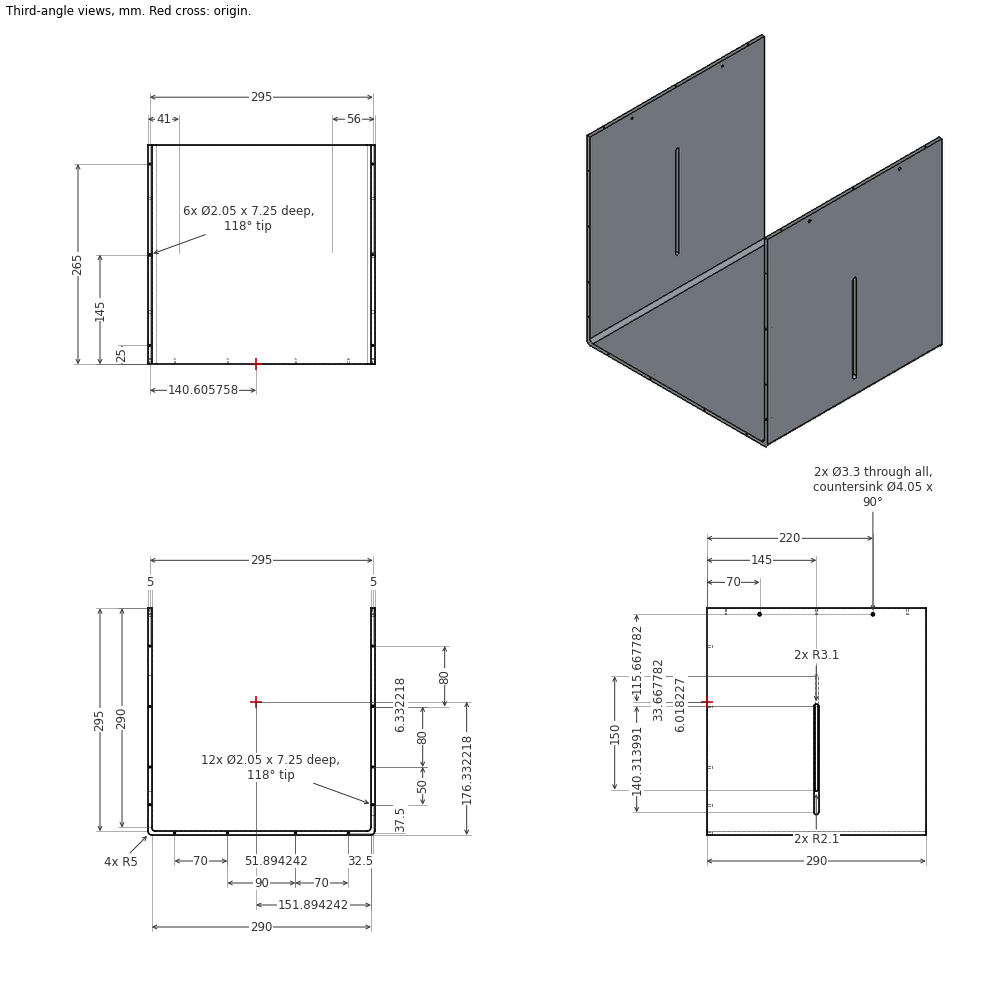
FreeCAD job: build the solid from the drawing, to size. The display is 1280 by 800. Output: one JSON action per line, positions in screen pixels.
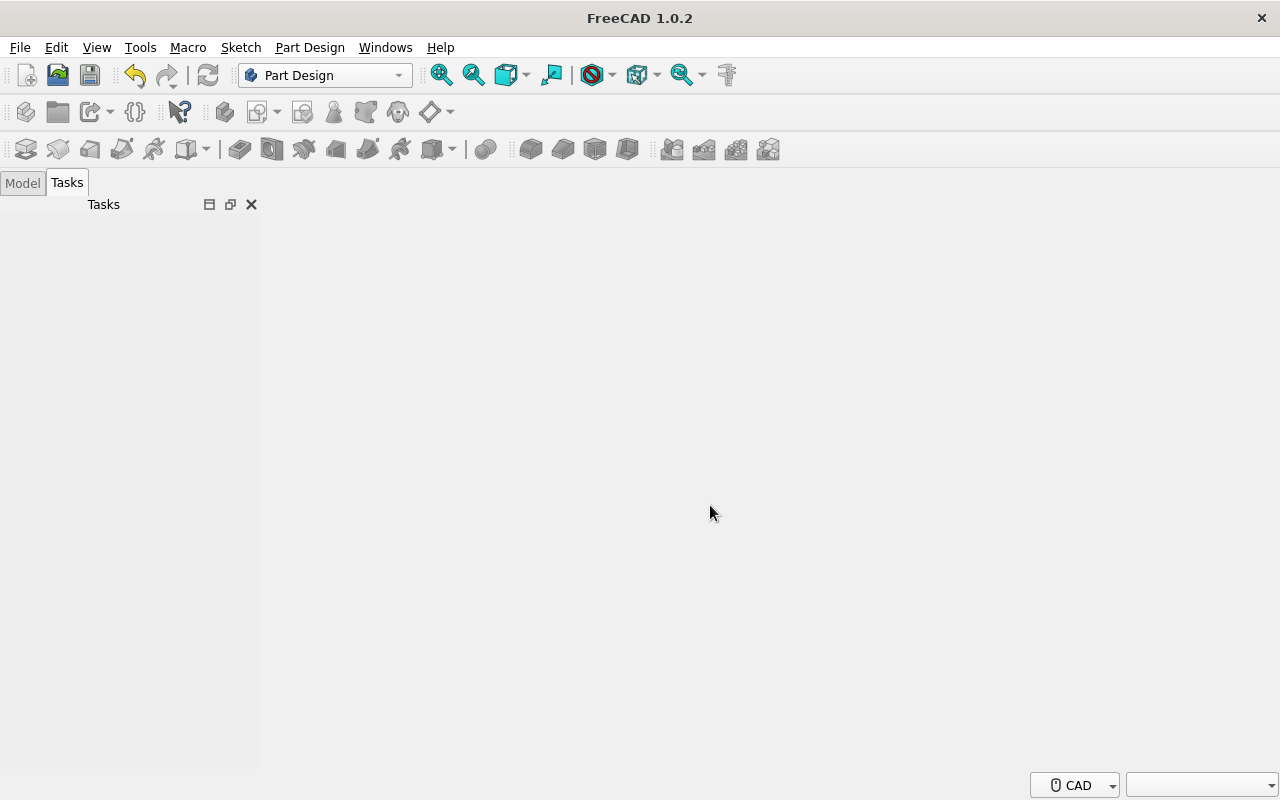
{"action": "left_click", "coordinate": [26, 76]}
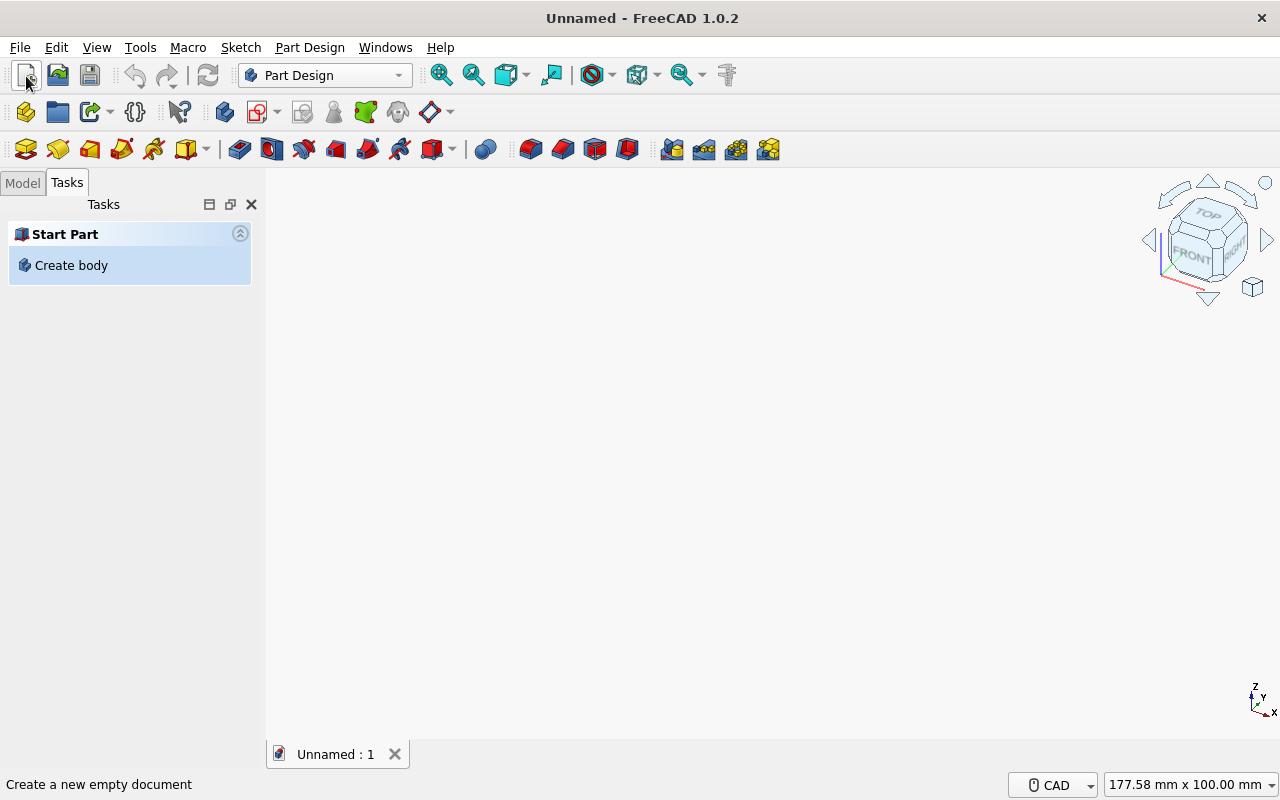
{"action": "left_click", "coordinate": [258, 112]}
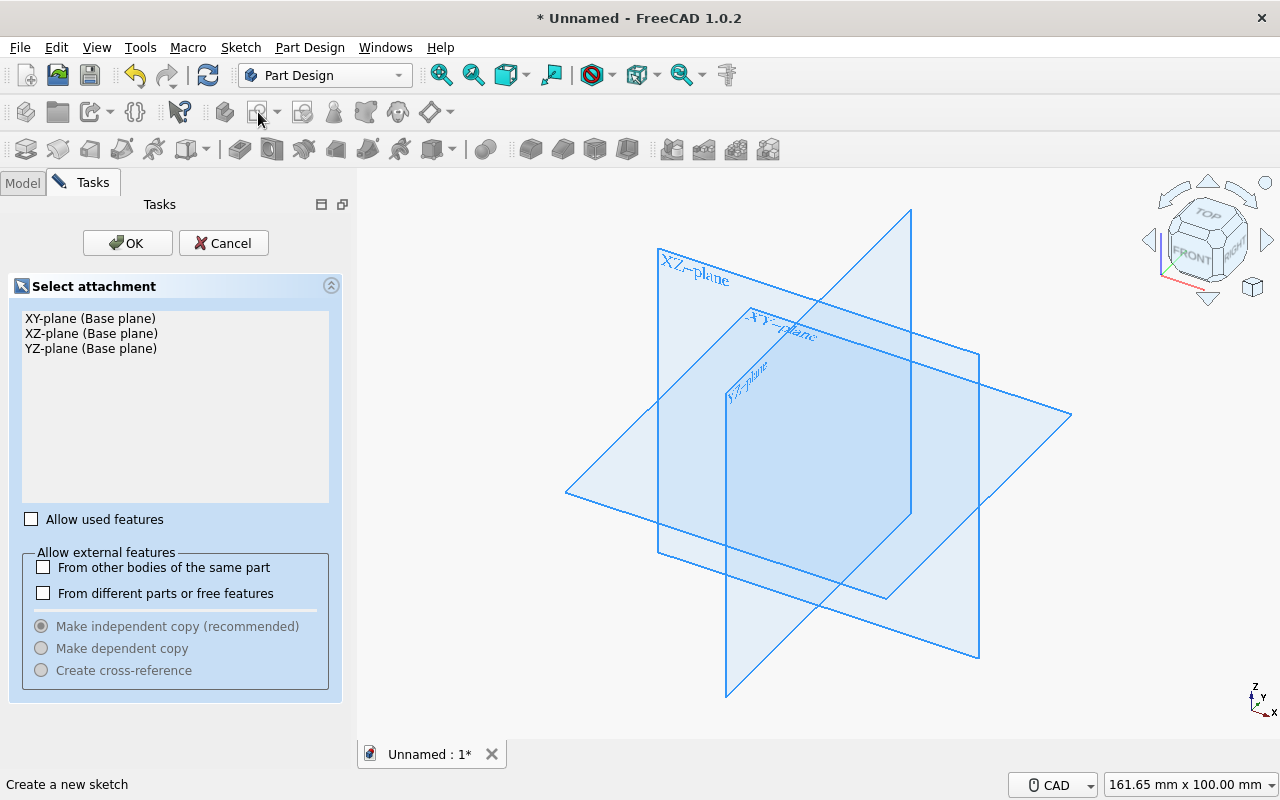
{"action": "left_click", "coordinate": [82, 334]}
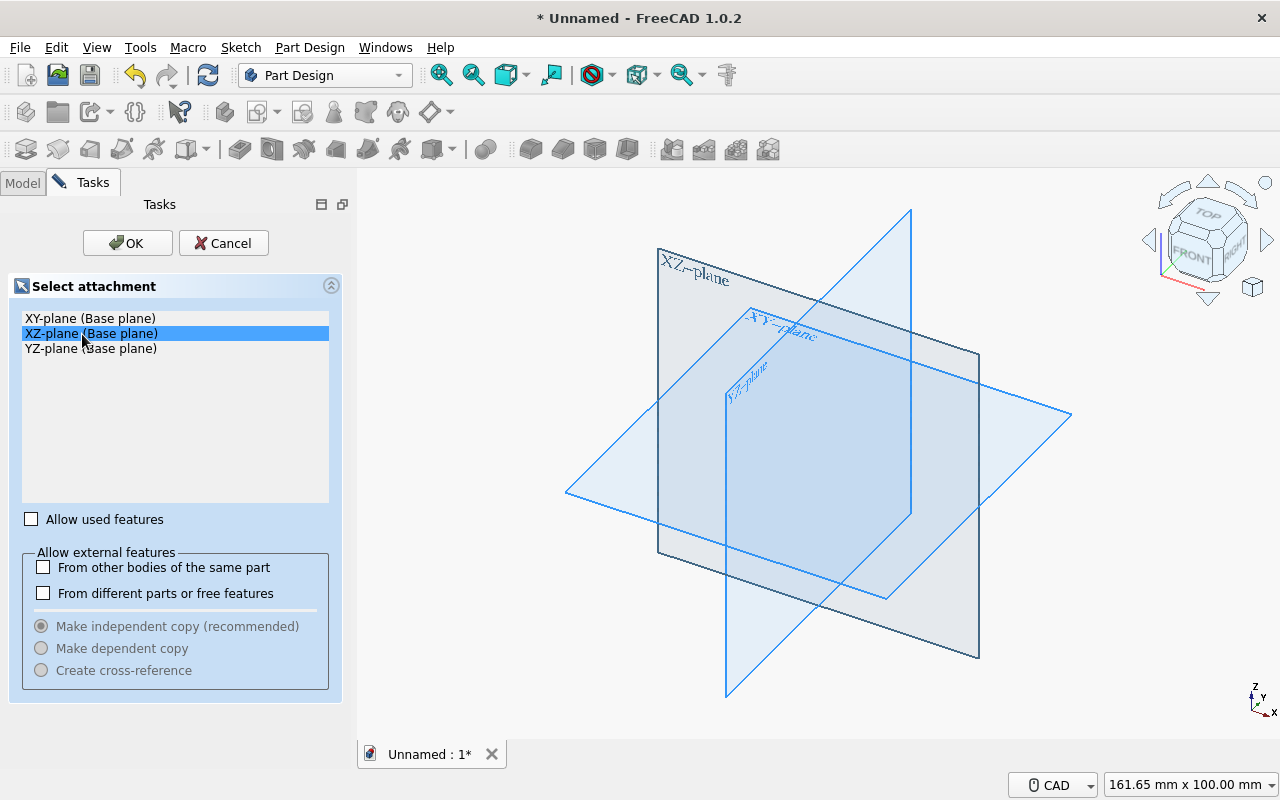
{"action": "left_click", "coordinate": [128, 243]}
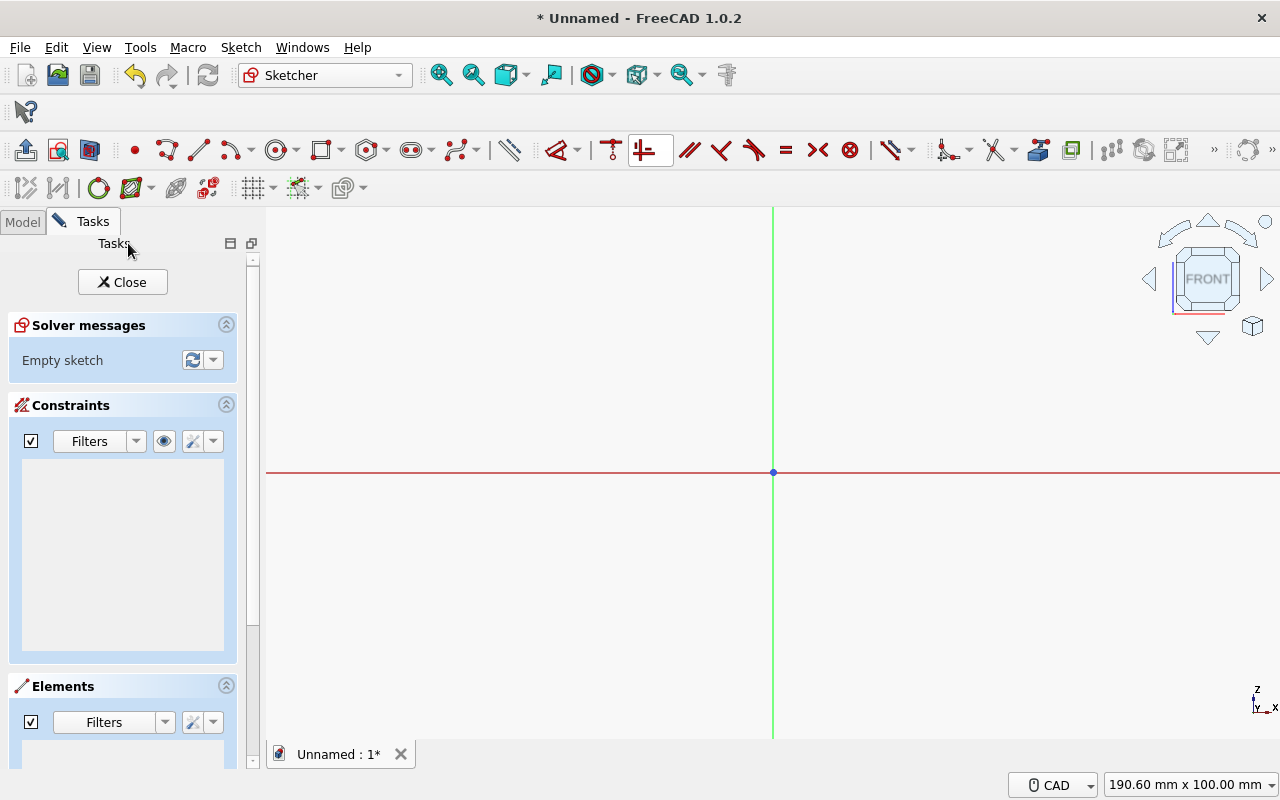
{"action": "scroll", "coordinate": [678, 438], "scroll_direction": "down", "scroll_amount": 8}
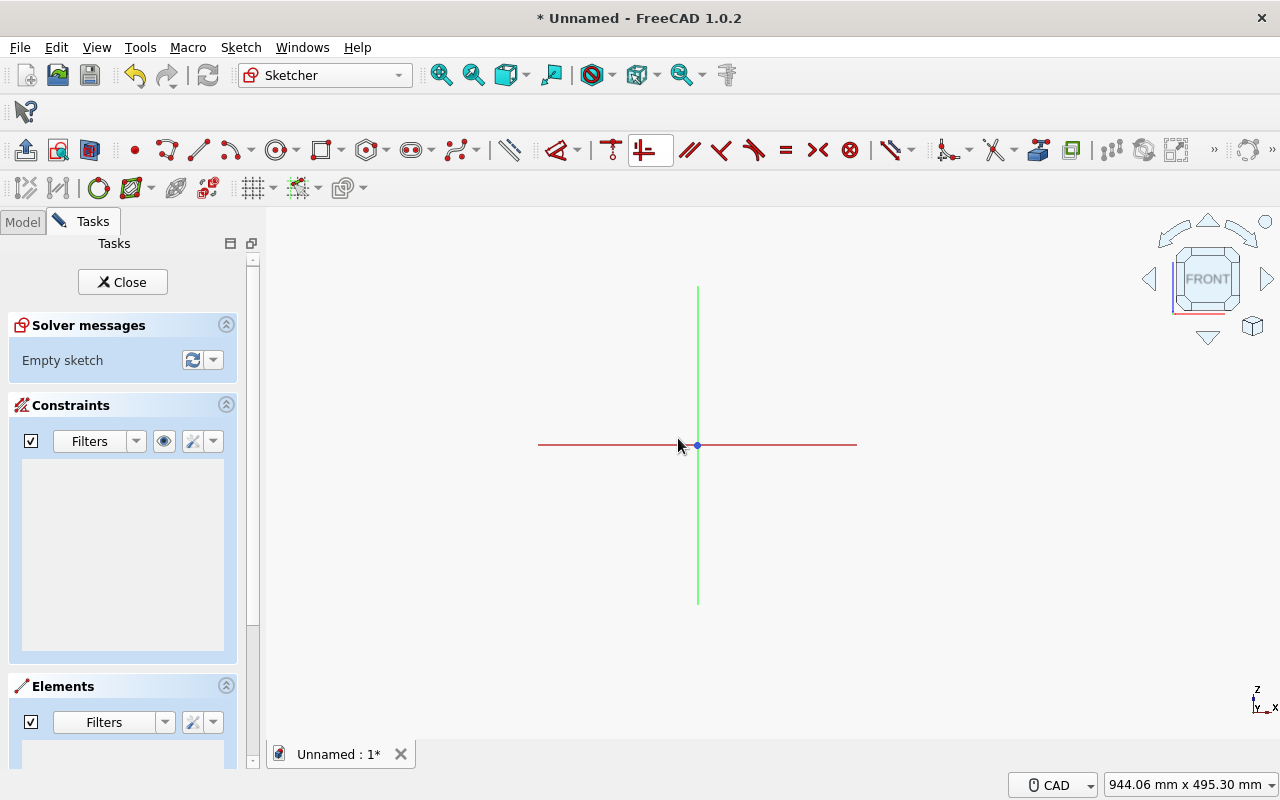
{"action": "left_click", "coordinate": [200, 150]}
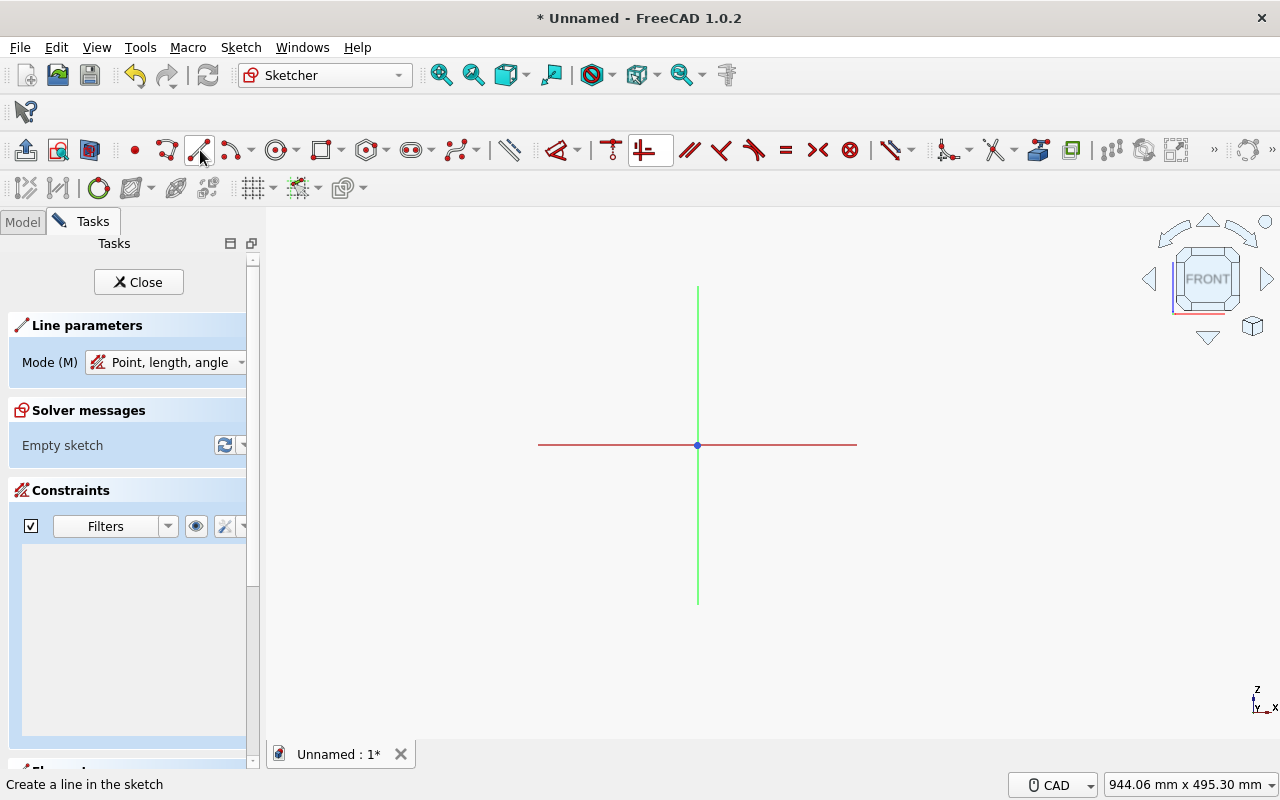
{"action": "left_click", "coordinate": [861, 635]}
{"action": "left_click", "coordinate": [549, 635]}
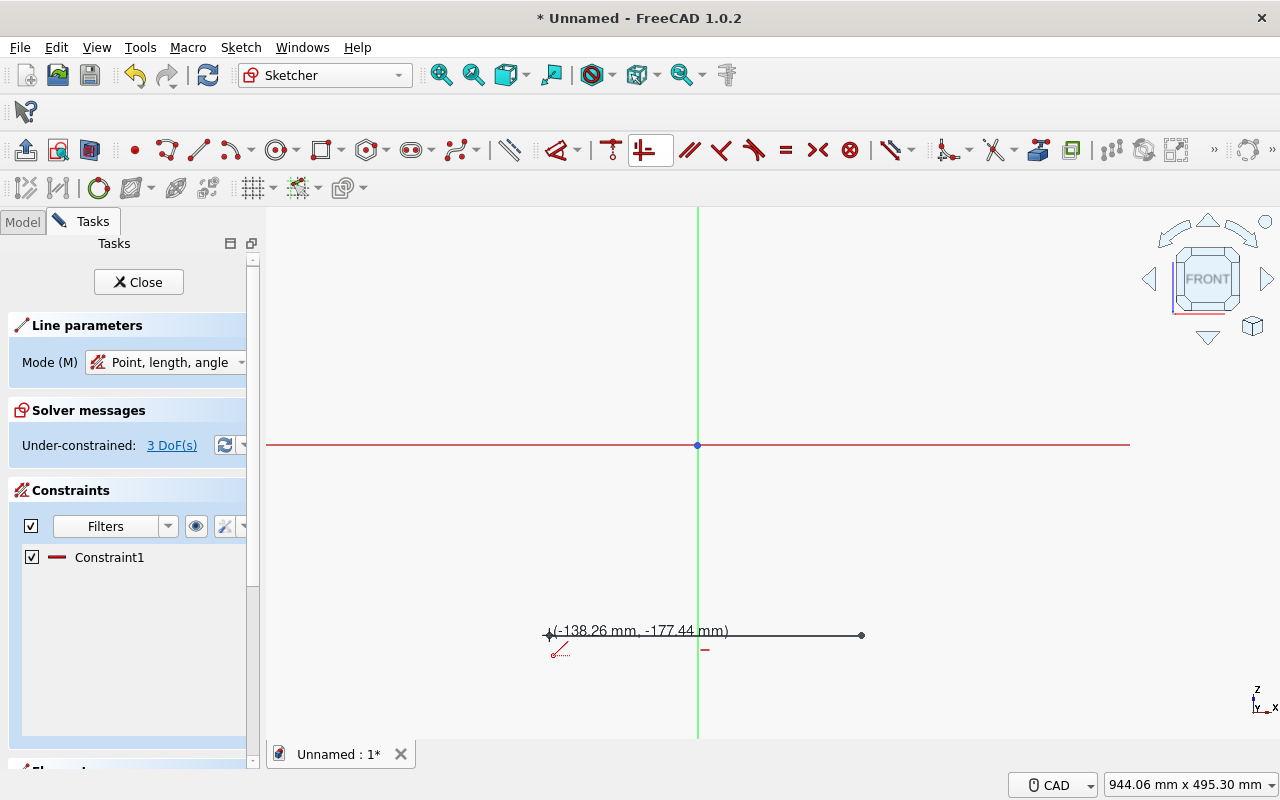
{"action": "left_click", "coordinate": [168, 150]}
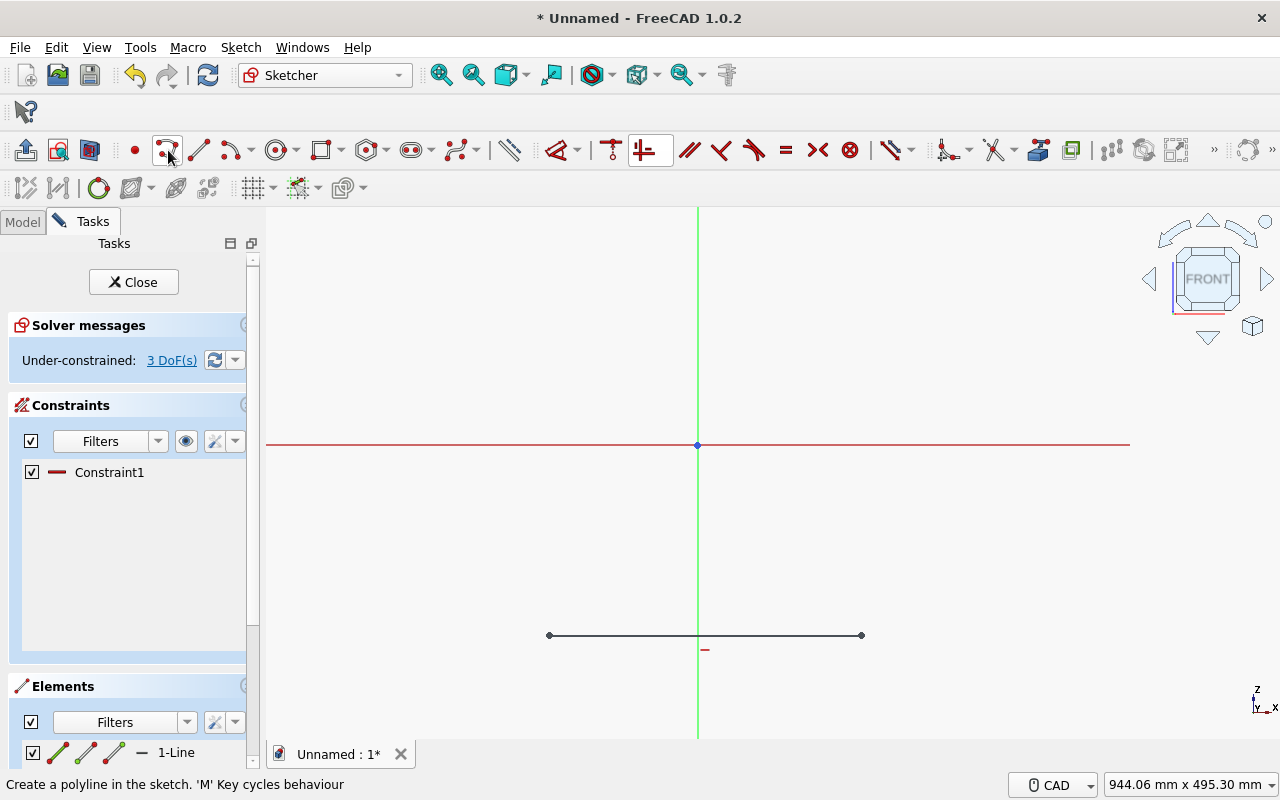
{"action": "scroll", "coordinate": [544, 629], "scroll_direction": "up", "scroll_amount": 4}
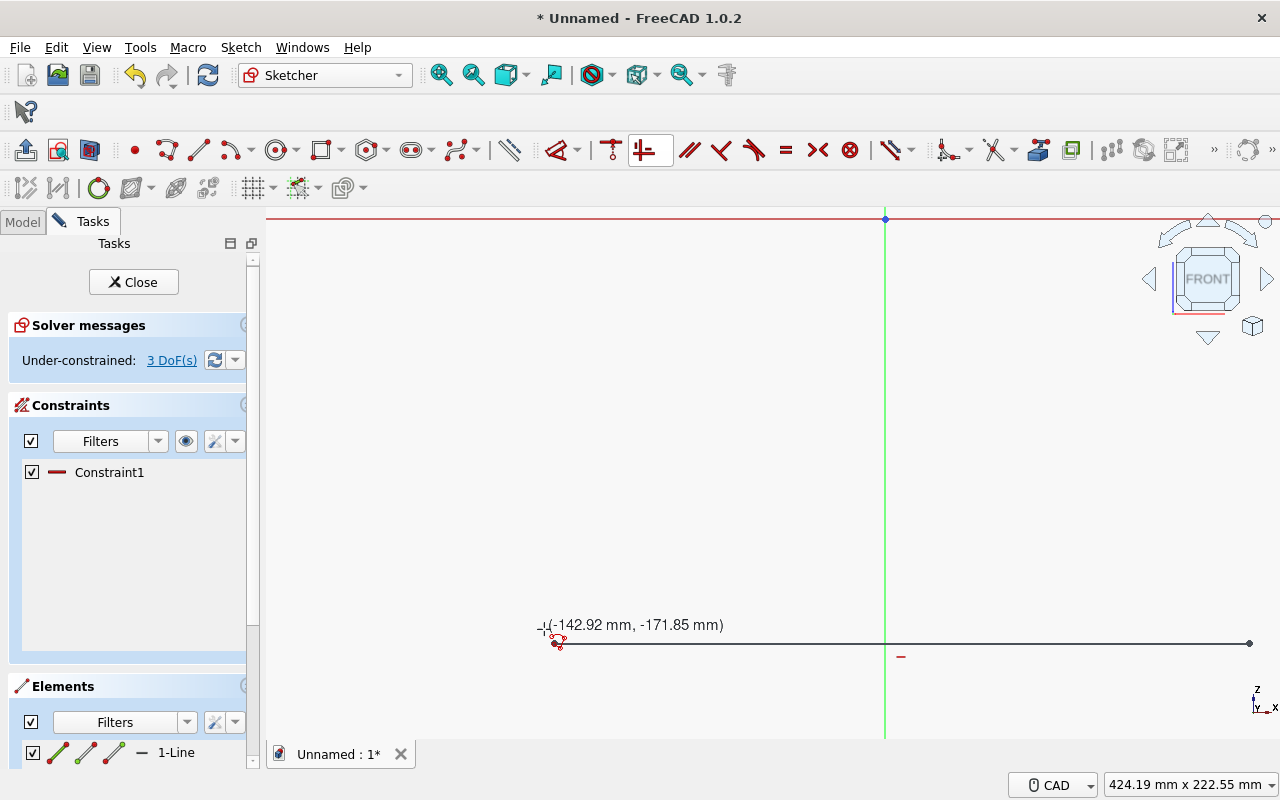
{"action": "left_click", "coordinate": [543, 629]}